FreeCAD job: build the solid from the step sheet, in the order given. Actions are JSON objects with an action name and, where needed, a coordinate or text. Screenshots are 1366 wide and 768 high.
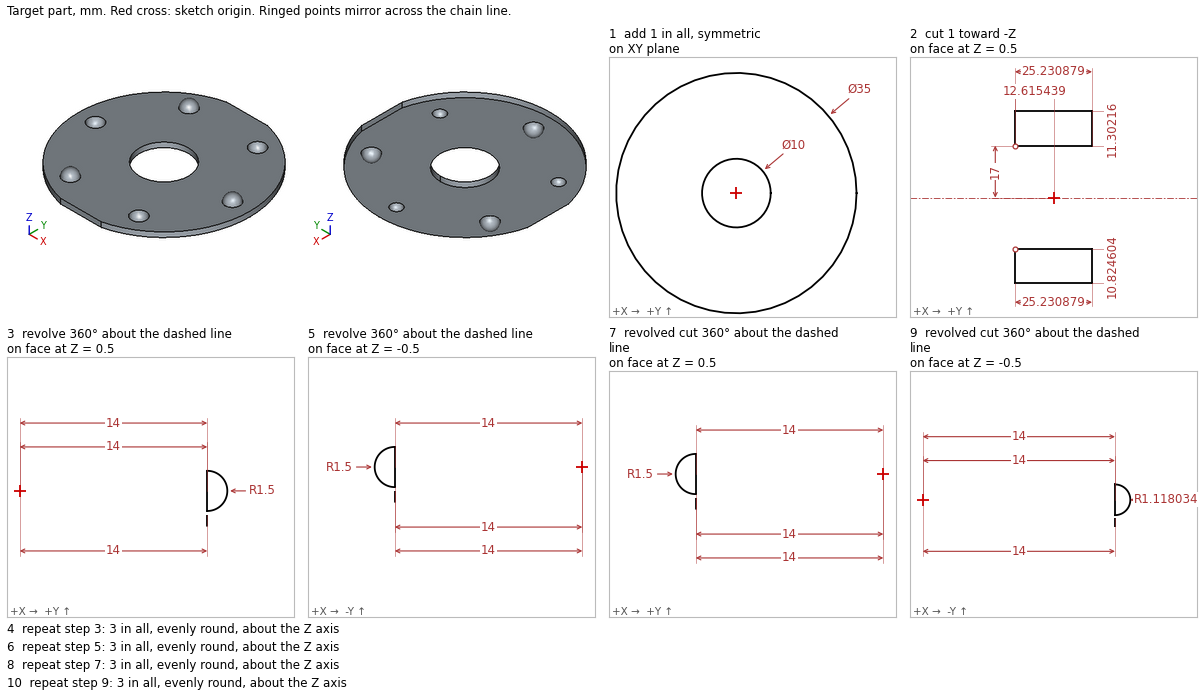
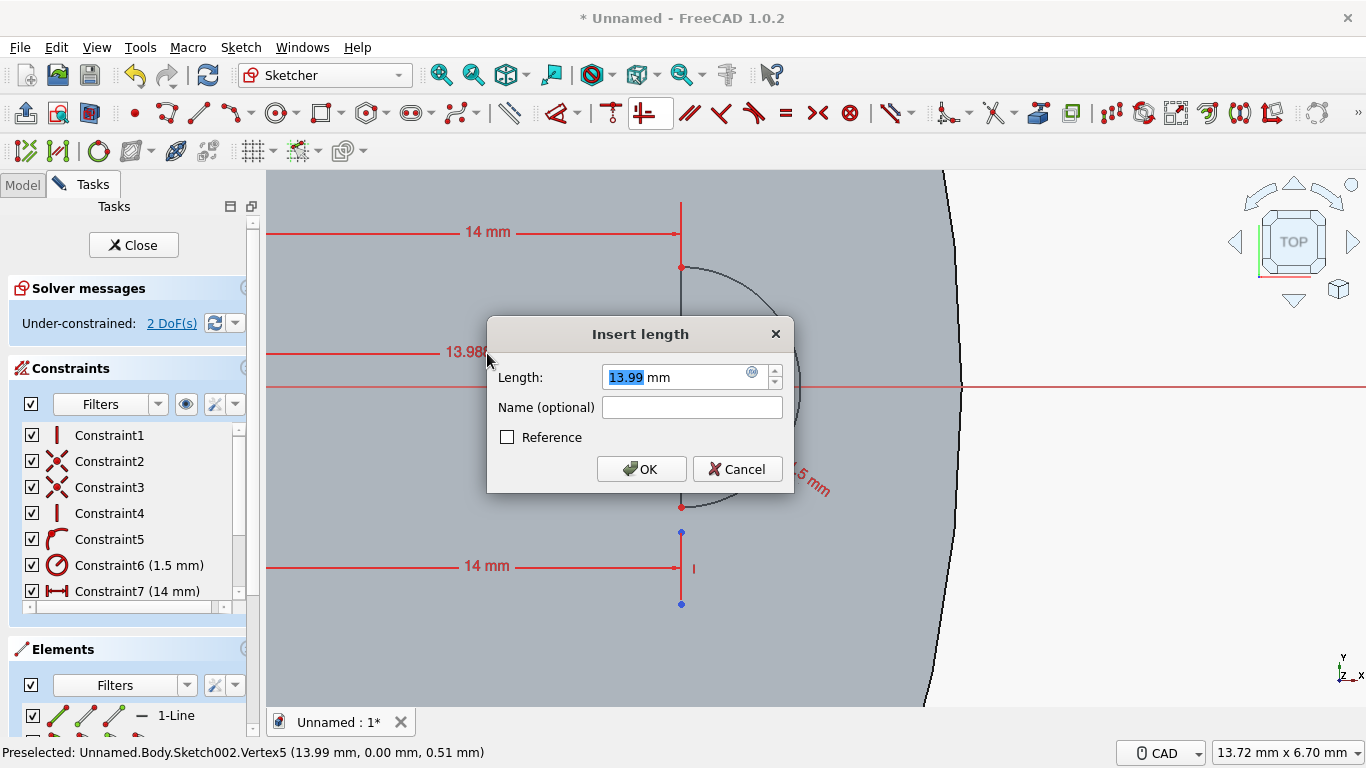
{"action": "type", "text": "14"}
{"action": "key", "text": "Return"}
{"action": "key", "text": "Escape"}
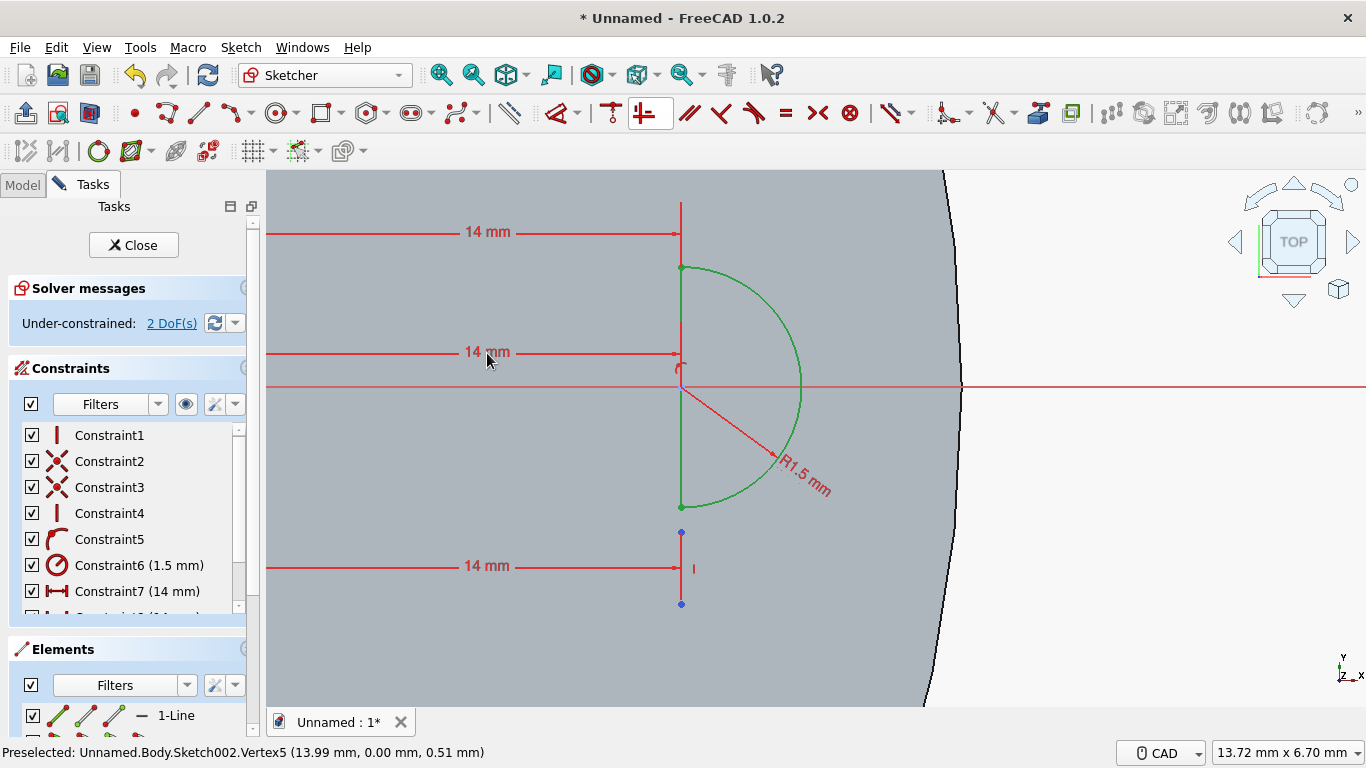
{"action": "left_click", "coordinate": [134, 245]}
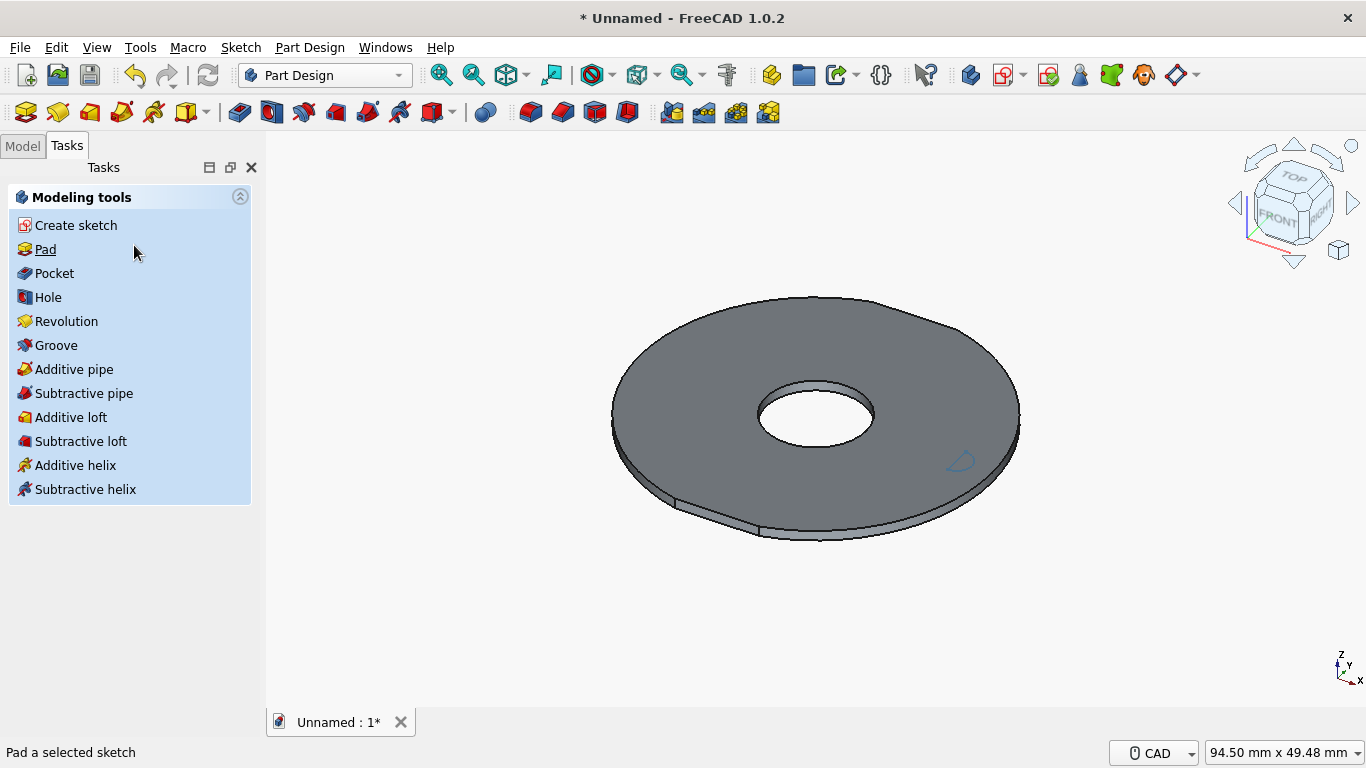
{"action": "left_click", "coordinate": [58, 112]}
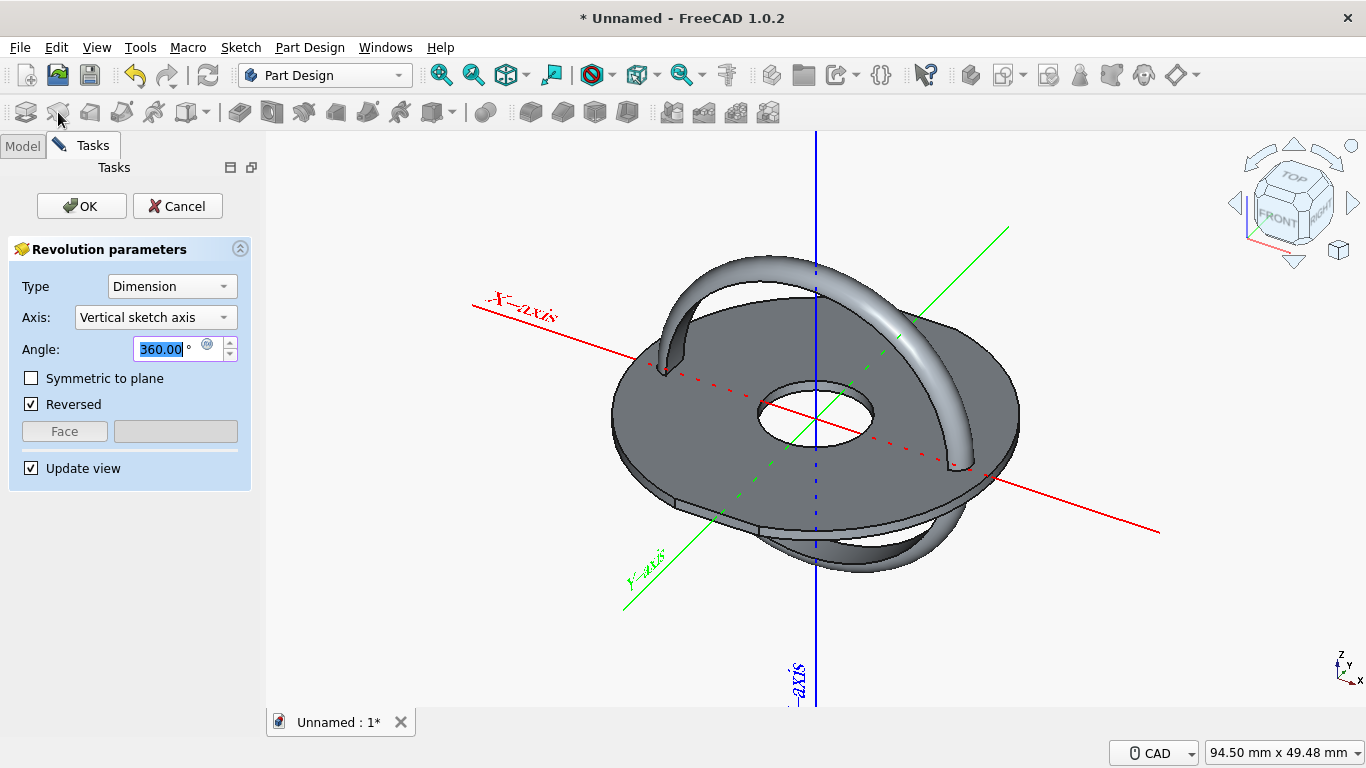
{"action": "left_click", "coordinate": [156, 318]}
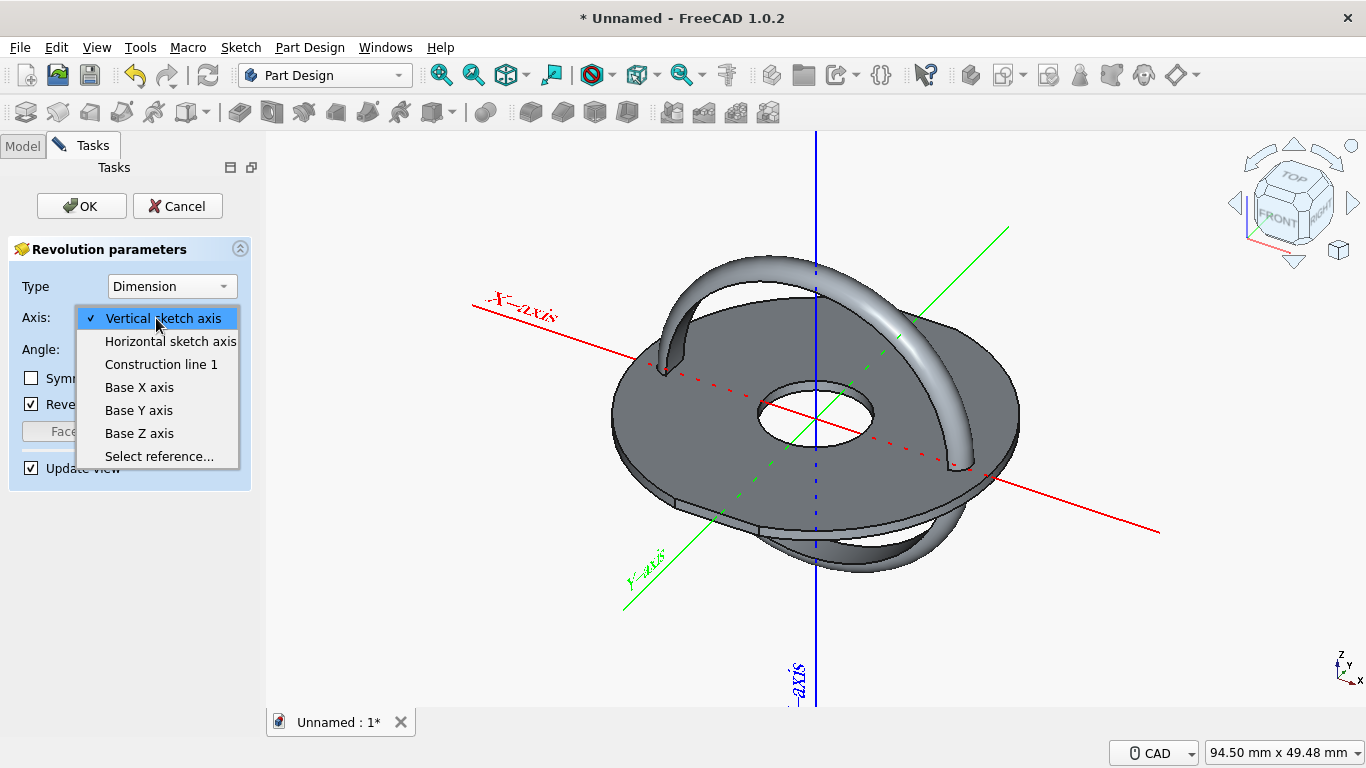
{"action": "left_click", "coordinate": [156, 364]}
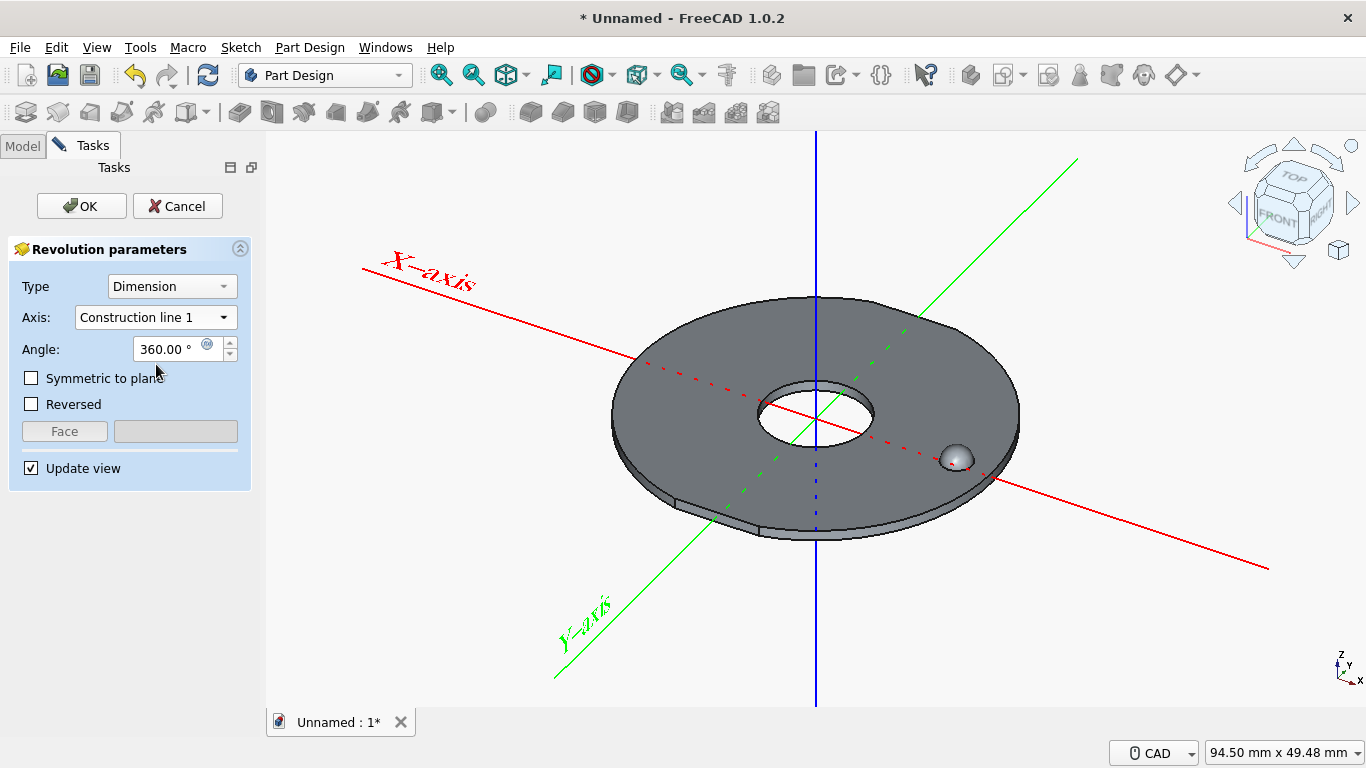
{"action": "left_click", "coordinate": [82, 206]}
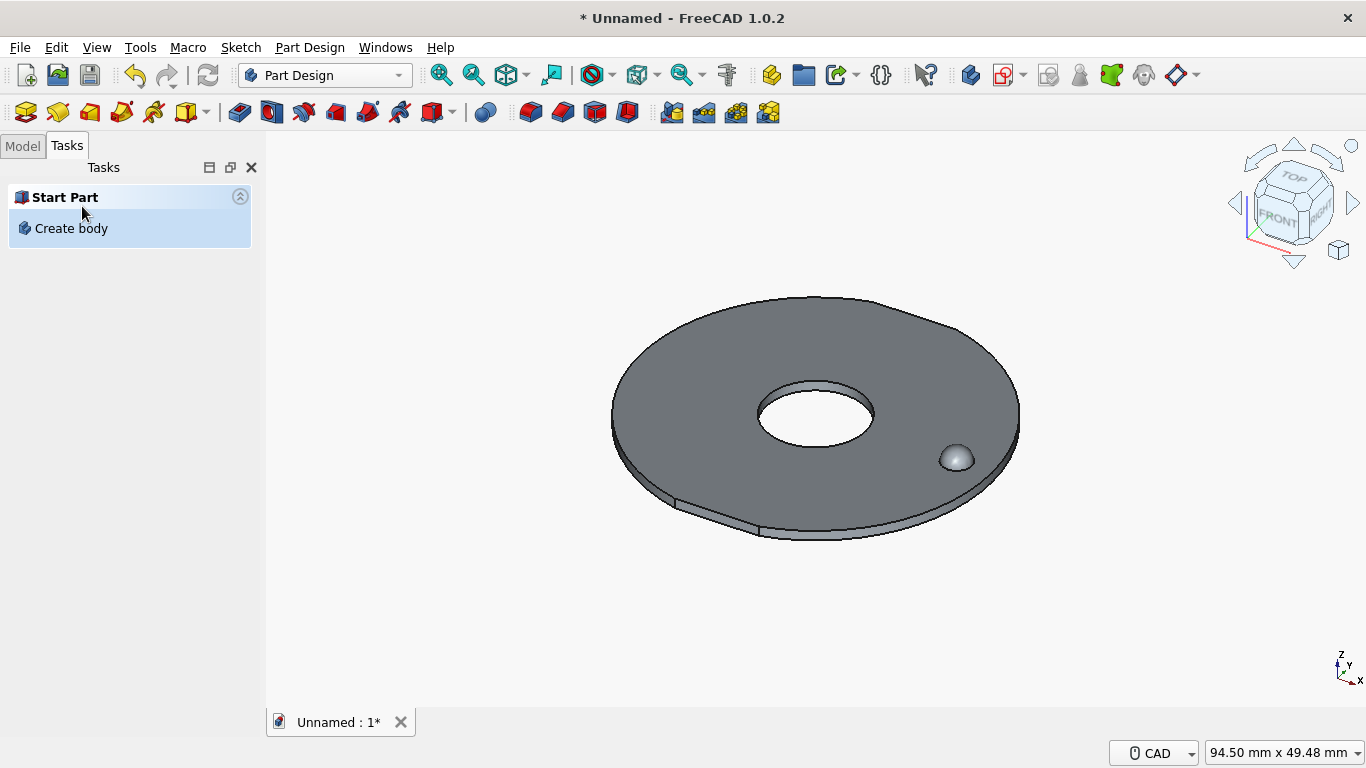
{"action": "left_click", "coordinate": [23, 145]}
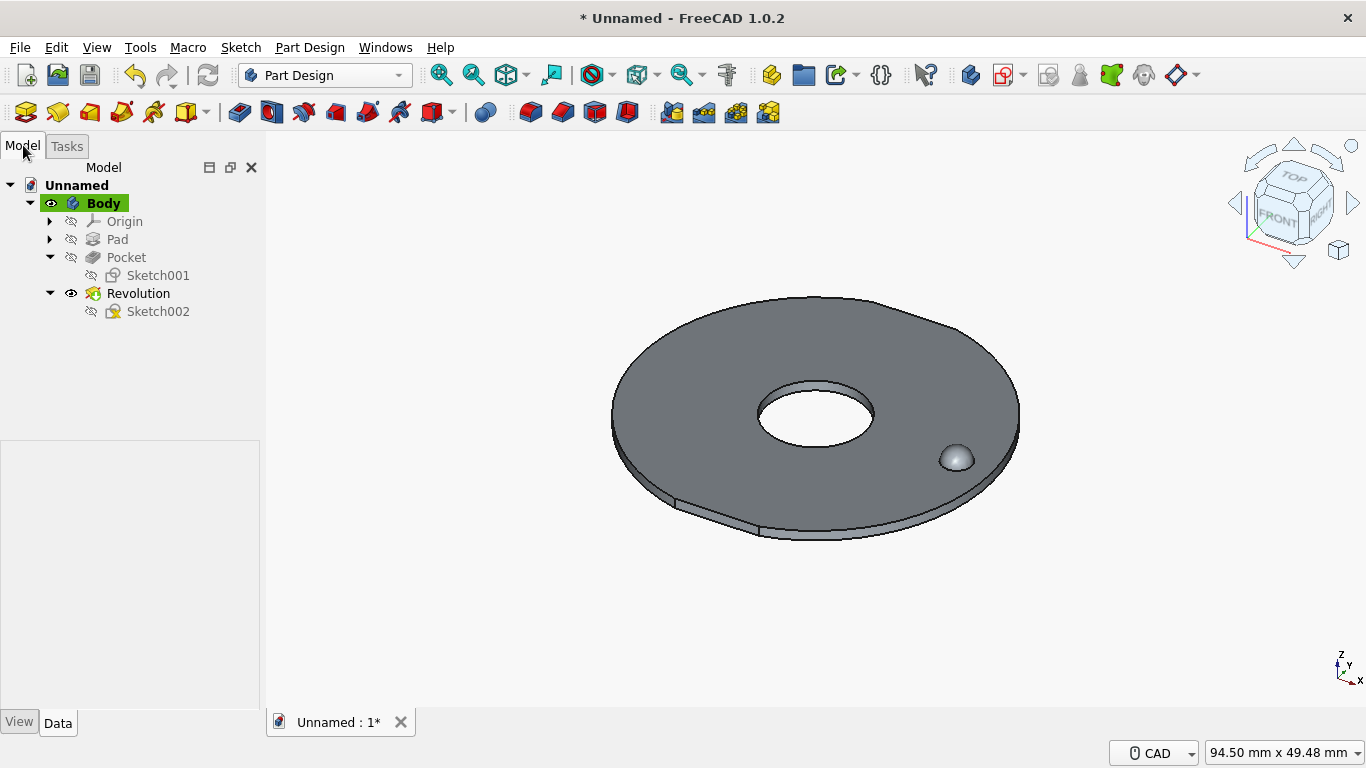
{"action": "left_click", "coordinate": [116, 293]}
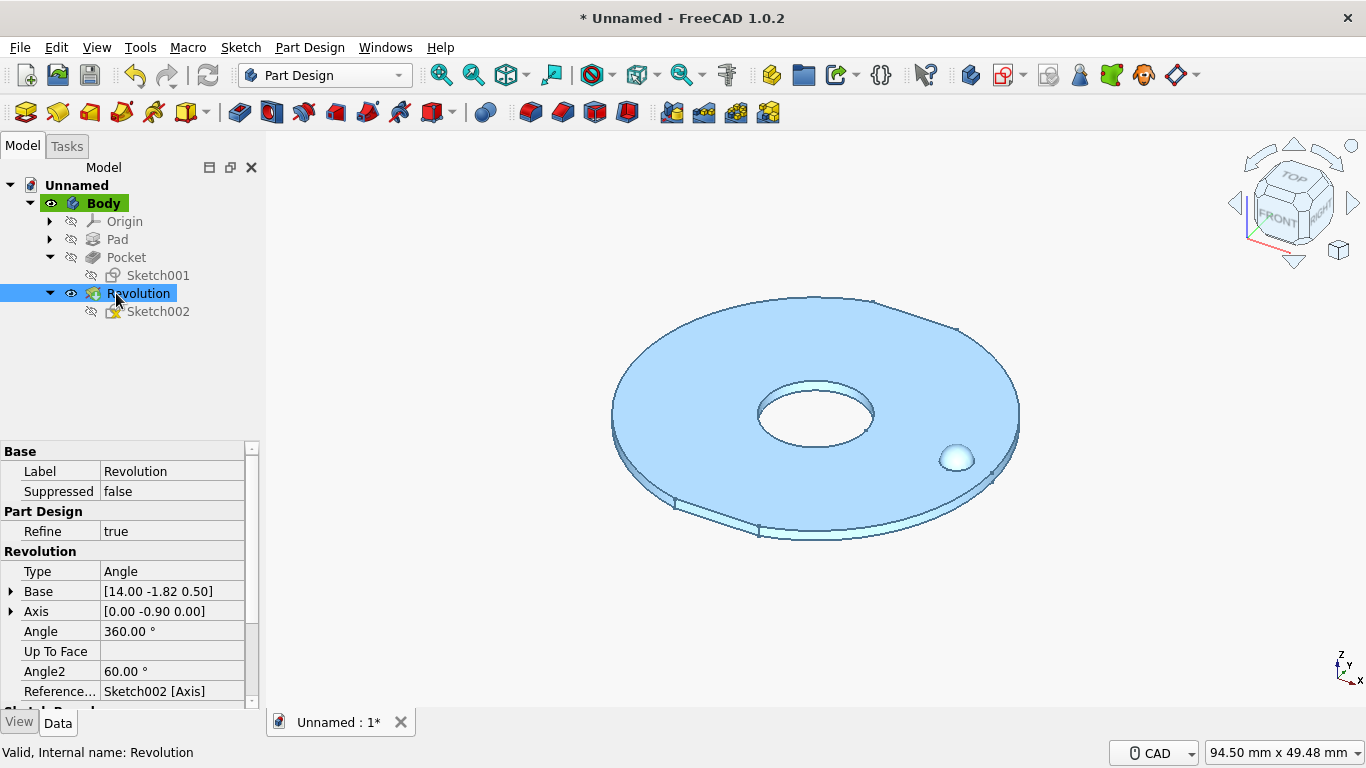
{"action": "left_click", "coordinate": [736, 112]}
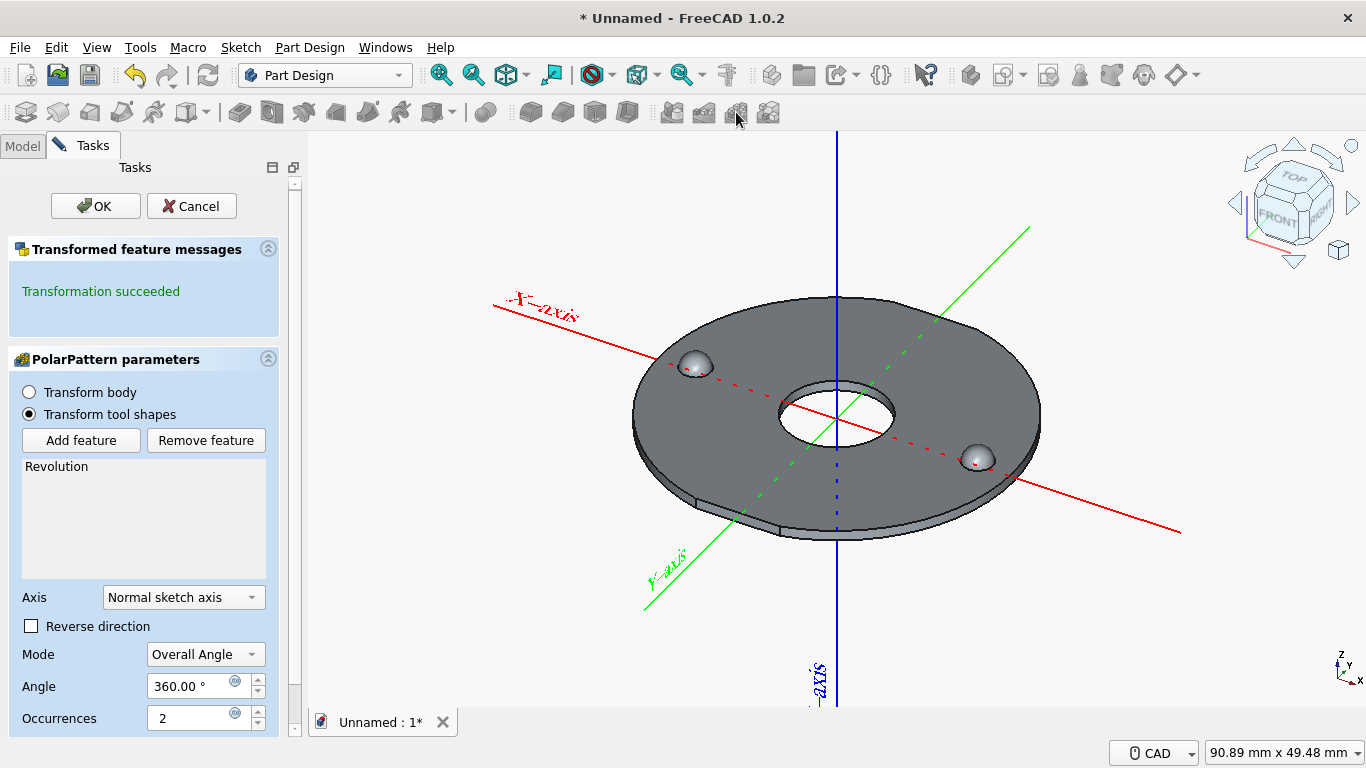
{"action": "left_click", "coordinate": [184, 598]}